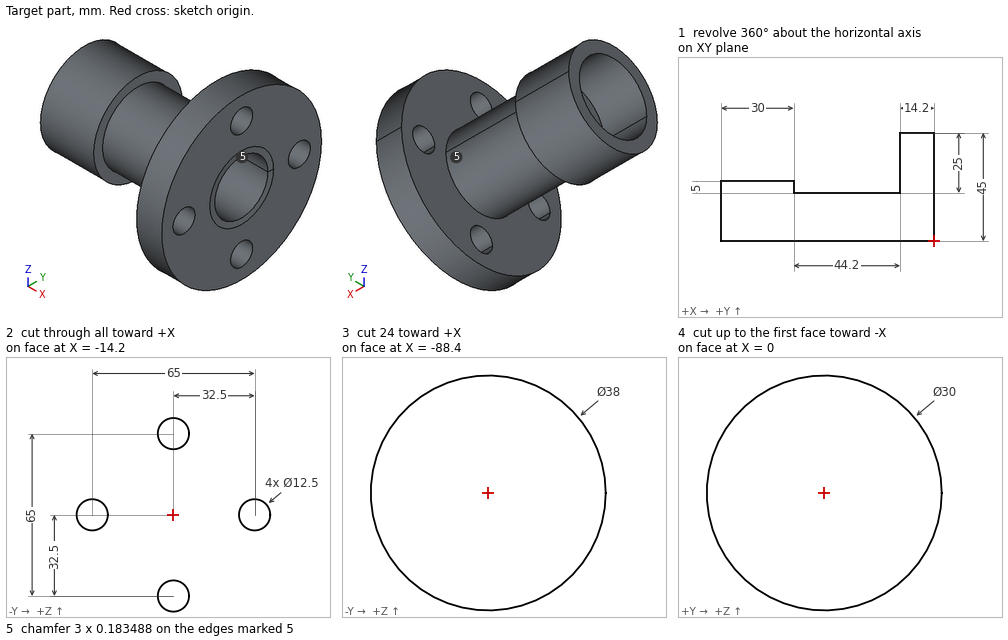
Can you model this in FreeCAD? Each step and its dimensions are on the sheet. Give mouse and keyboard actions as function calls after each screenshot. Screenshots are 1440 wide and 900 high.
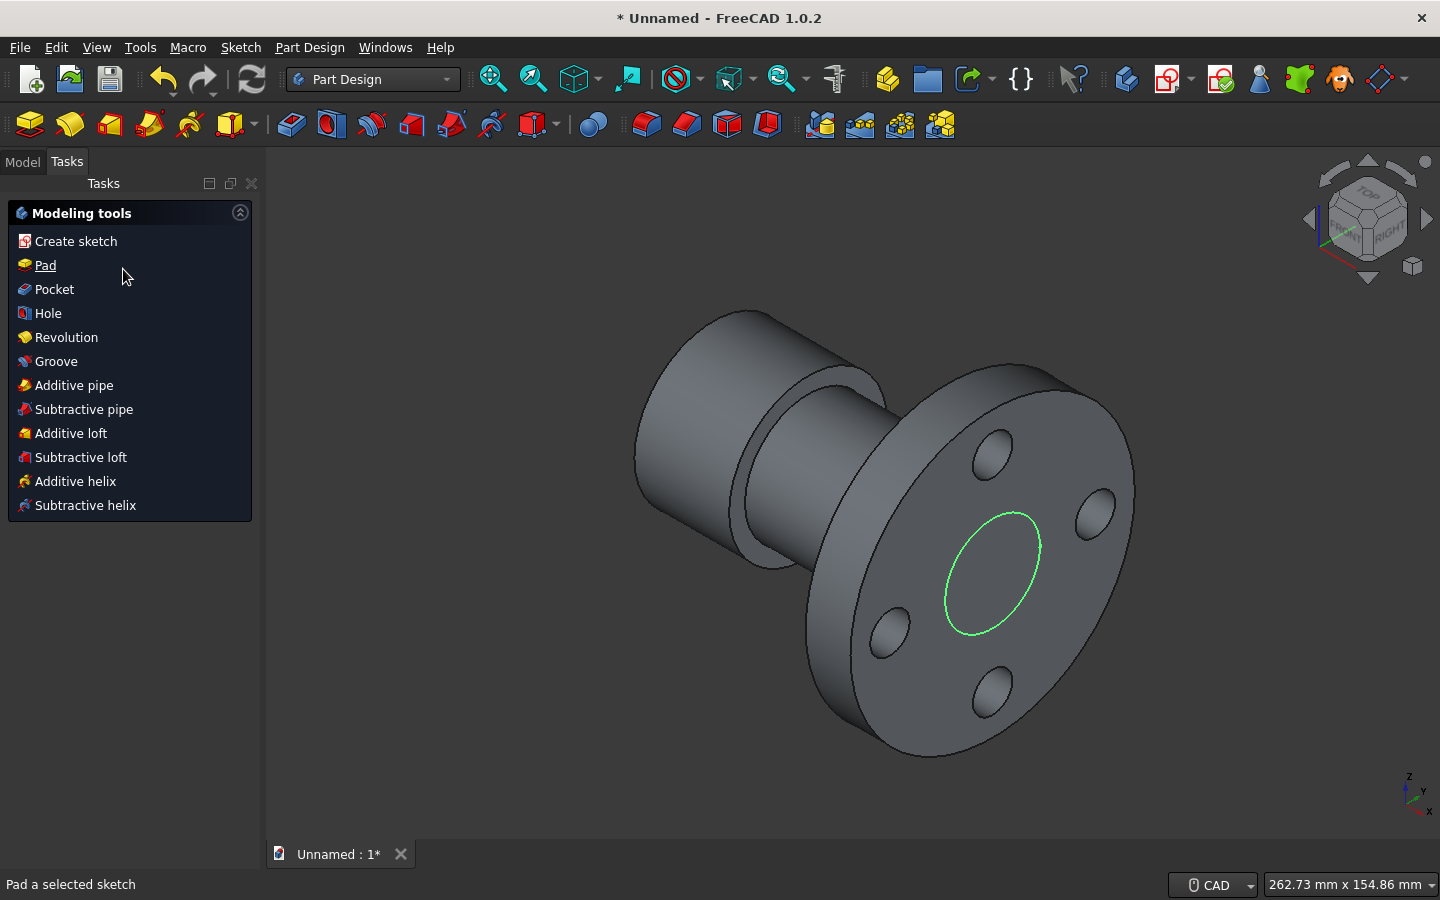
click(292, 124)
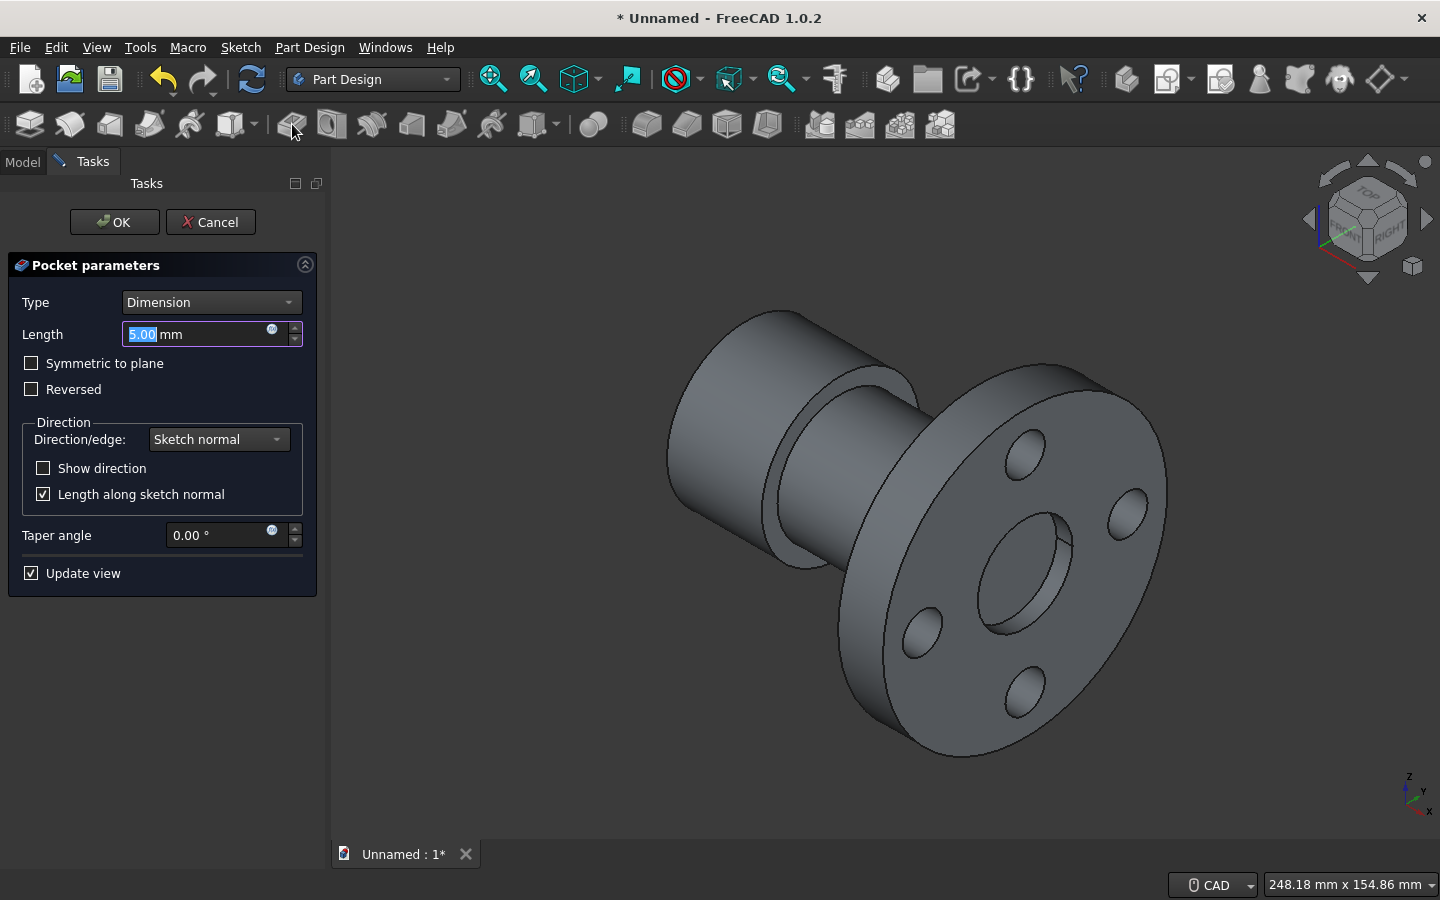
click(212, 302)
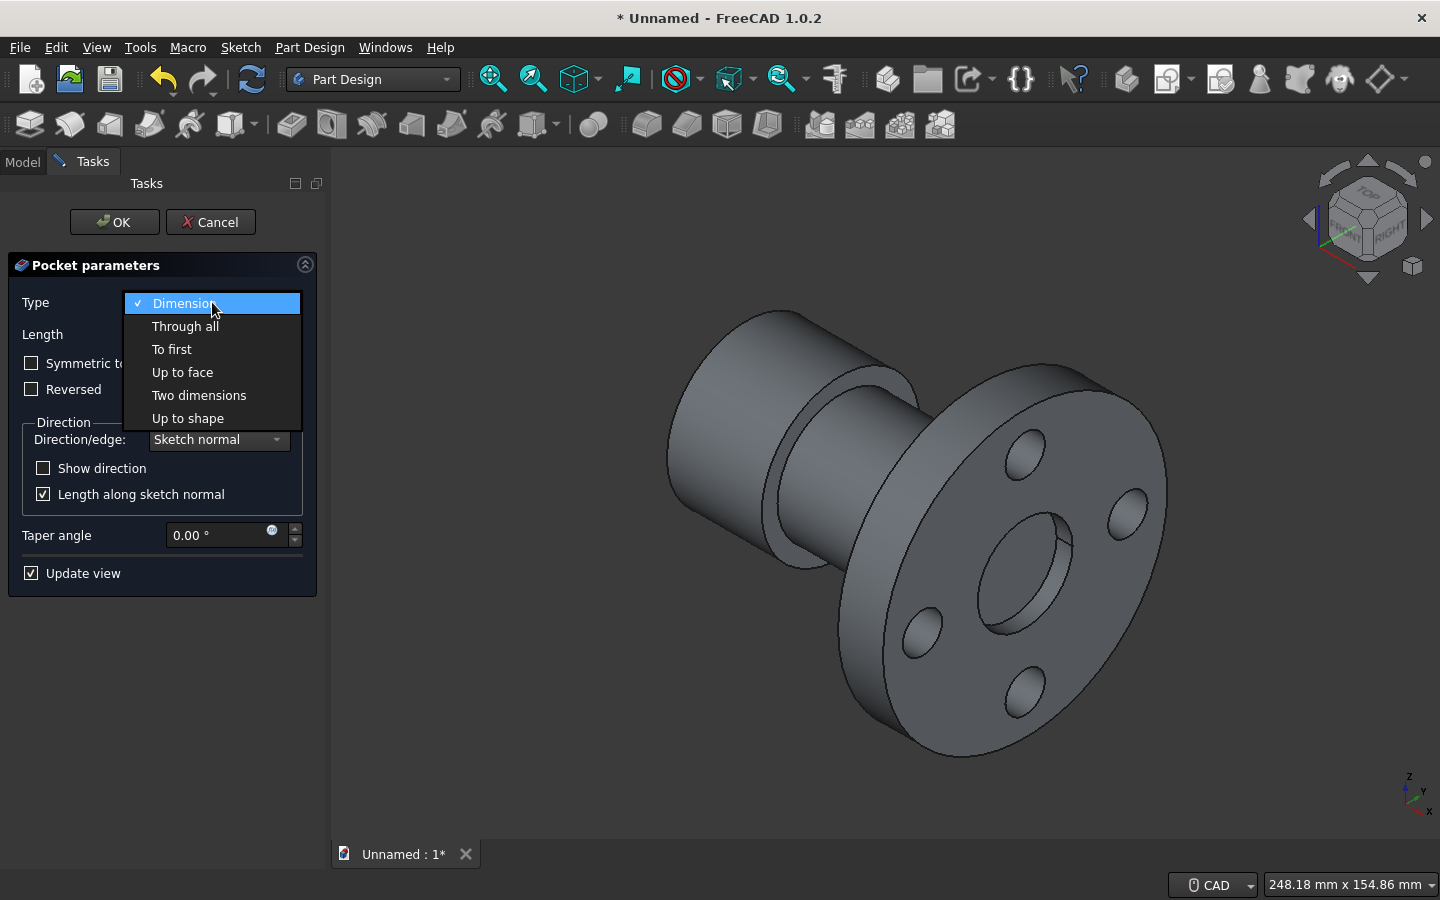
click(212, 350)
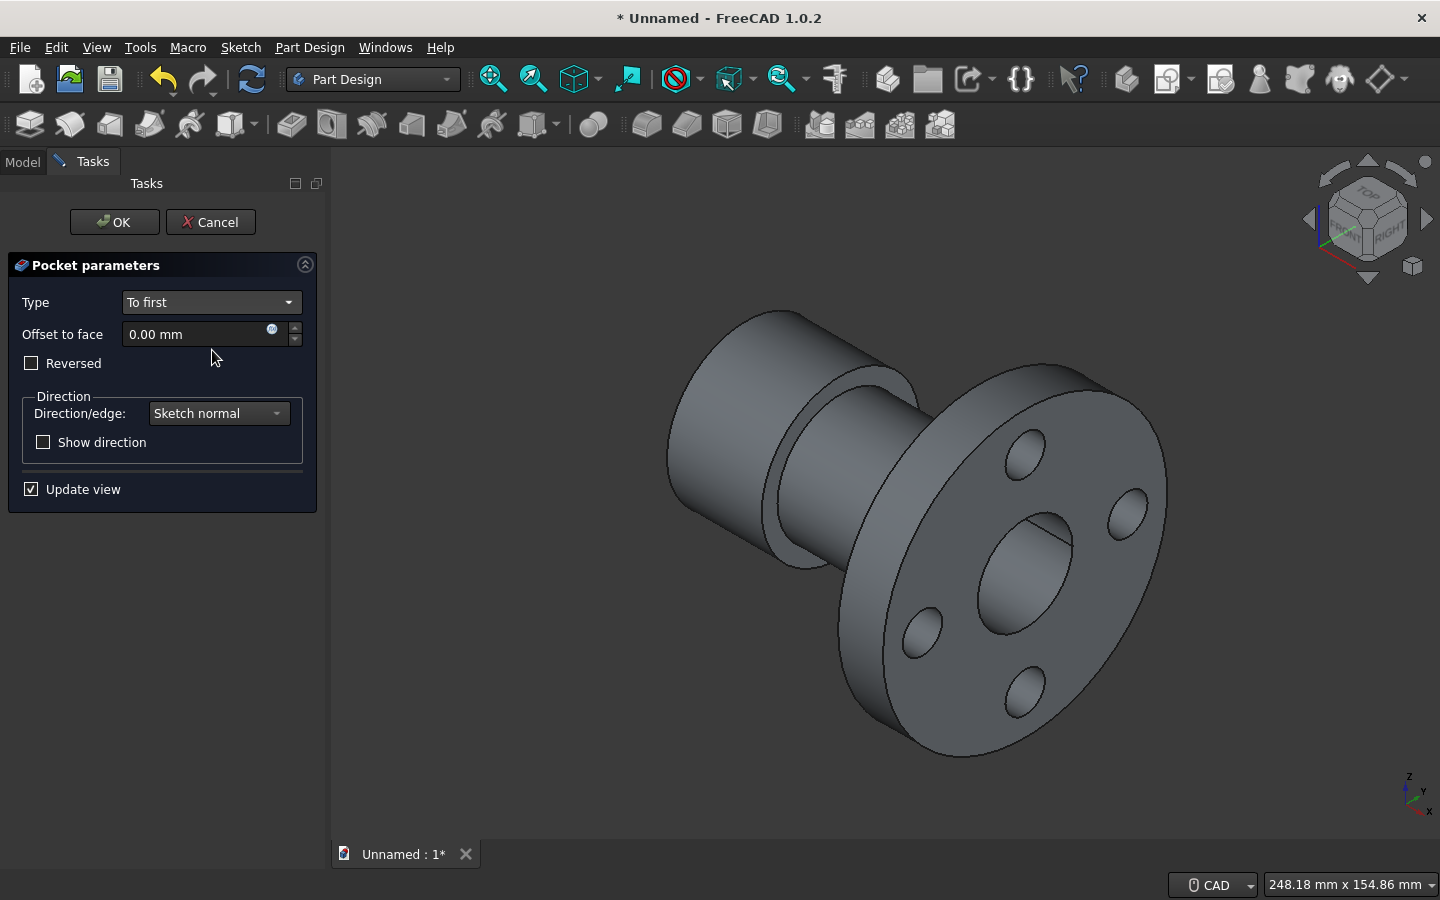
click(115, 222)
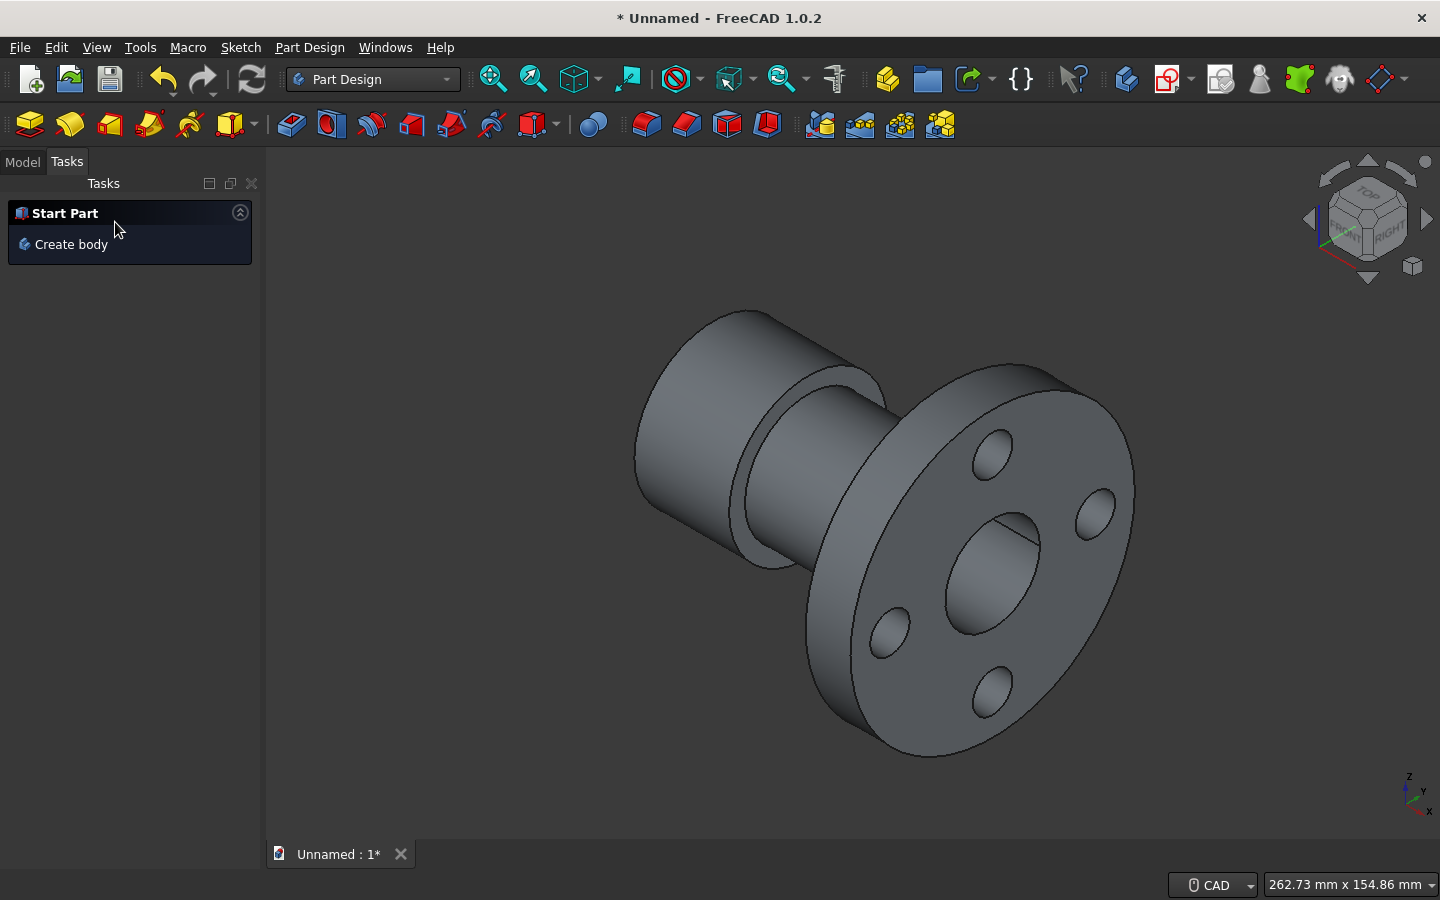
click(978, 633)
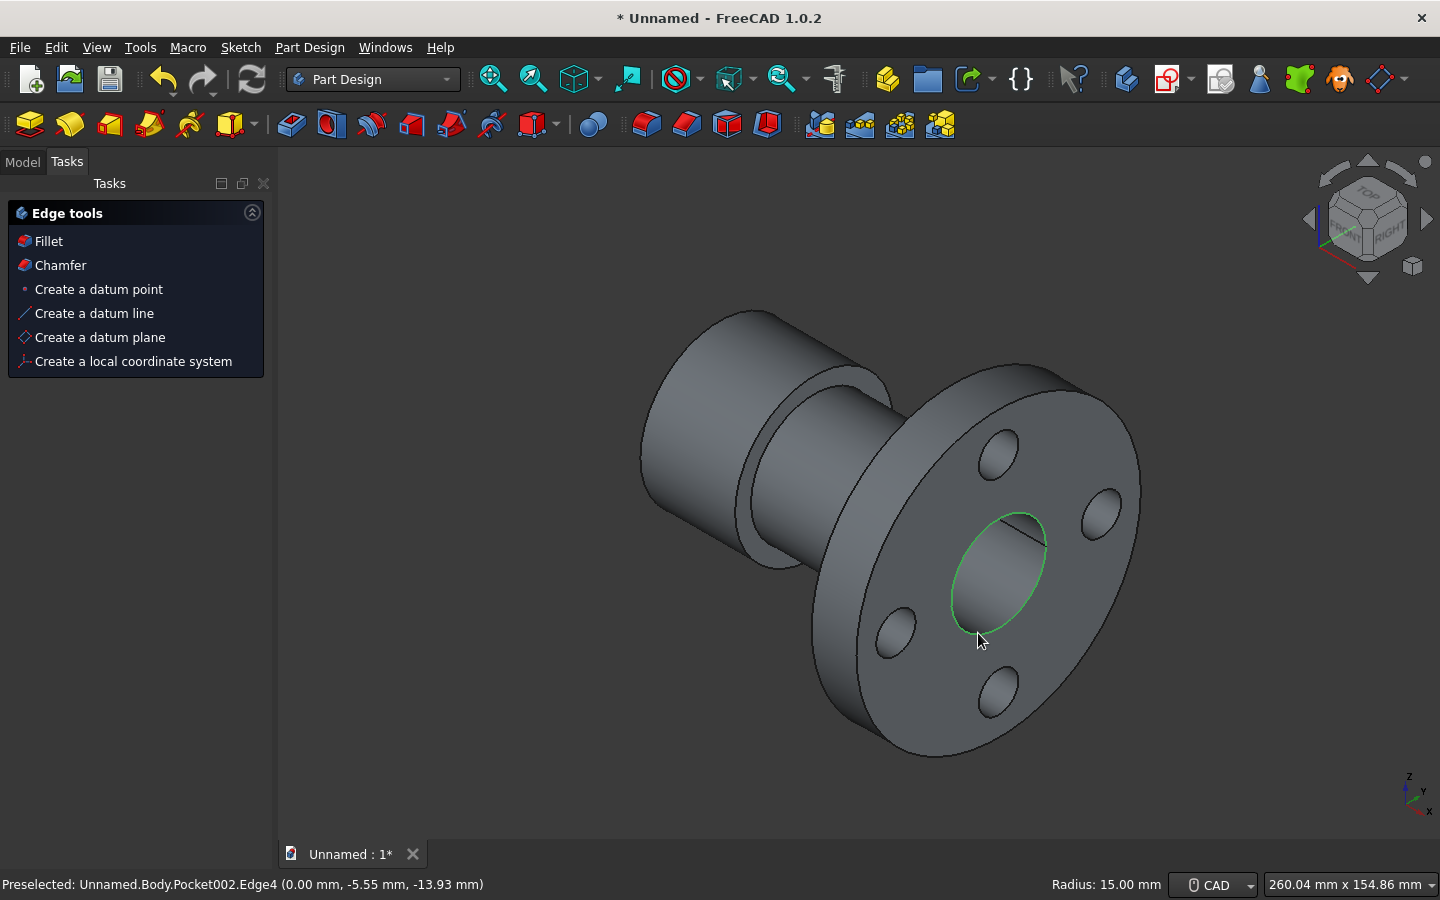
click(688, 124)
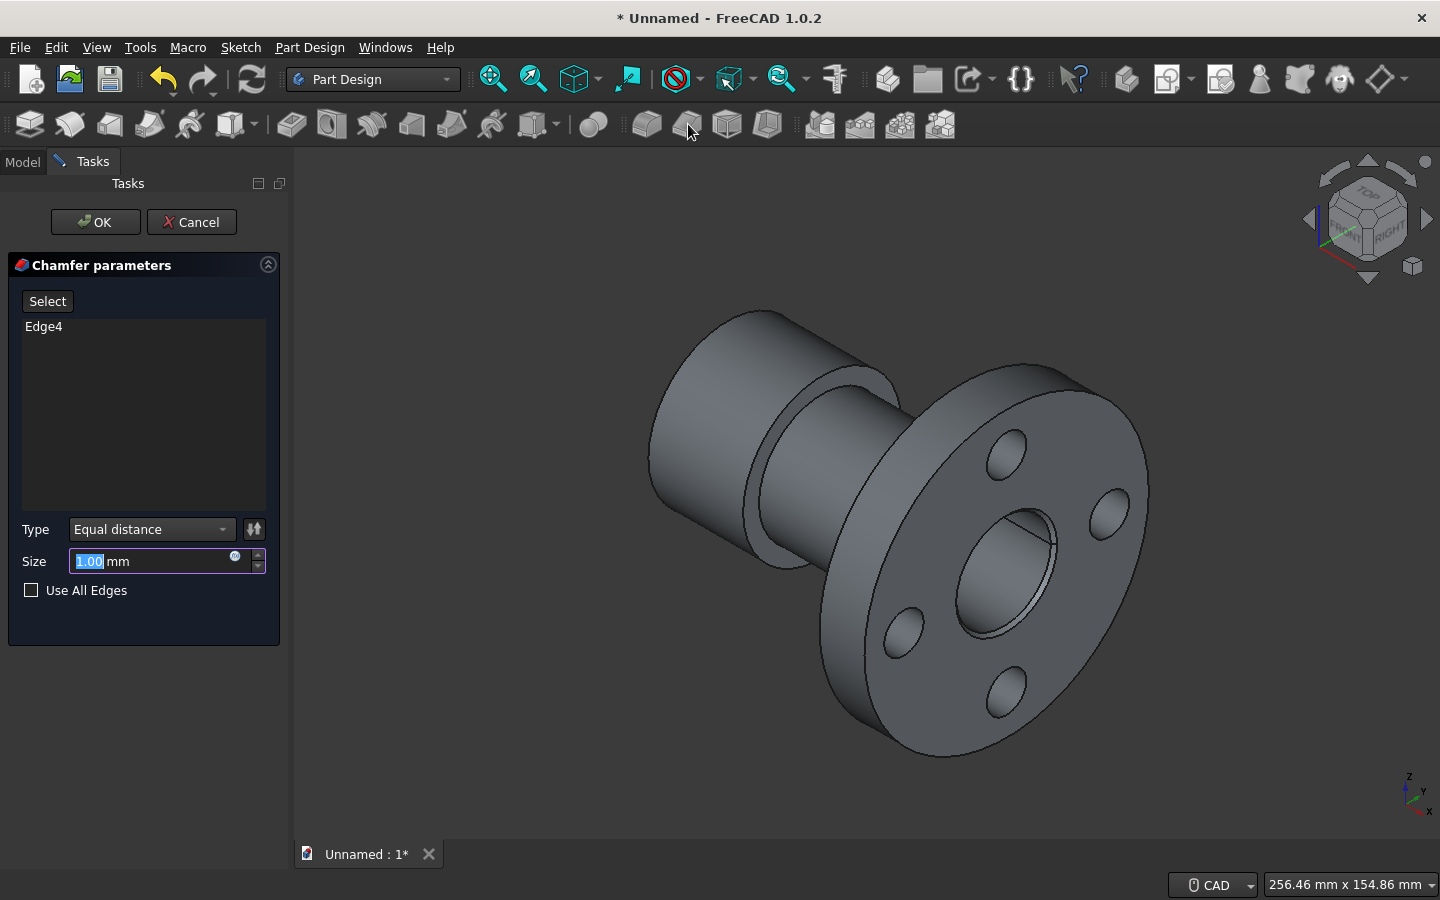
text(3)
key(Tab)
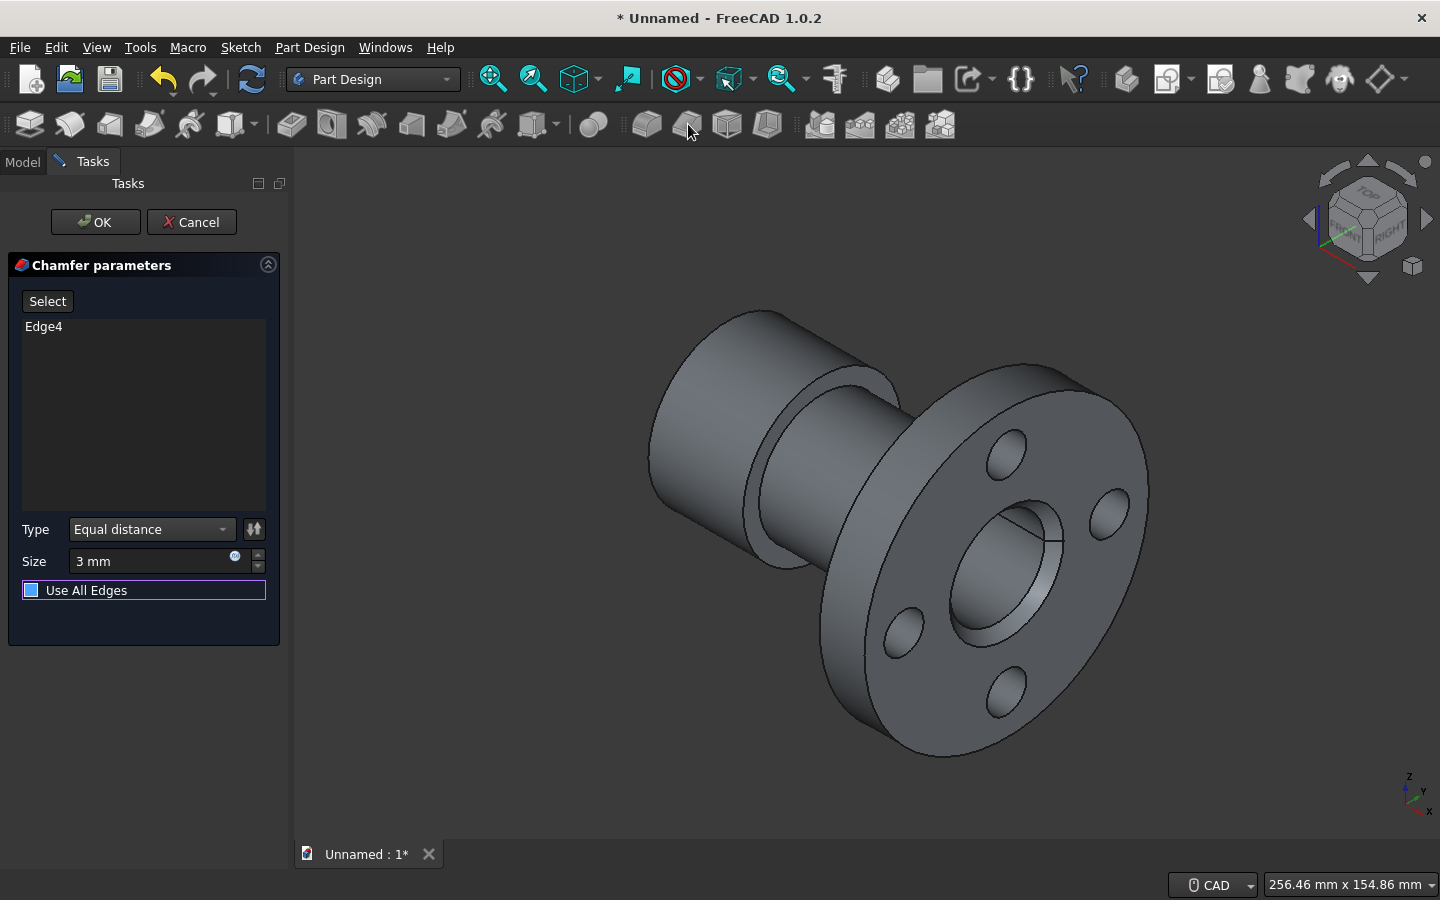
click(153, 530)